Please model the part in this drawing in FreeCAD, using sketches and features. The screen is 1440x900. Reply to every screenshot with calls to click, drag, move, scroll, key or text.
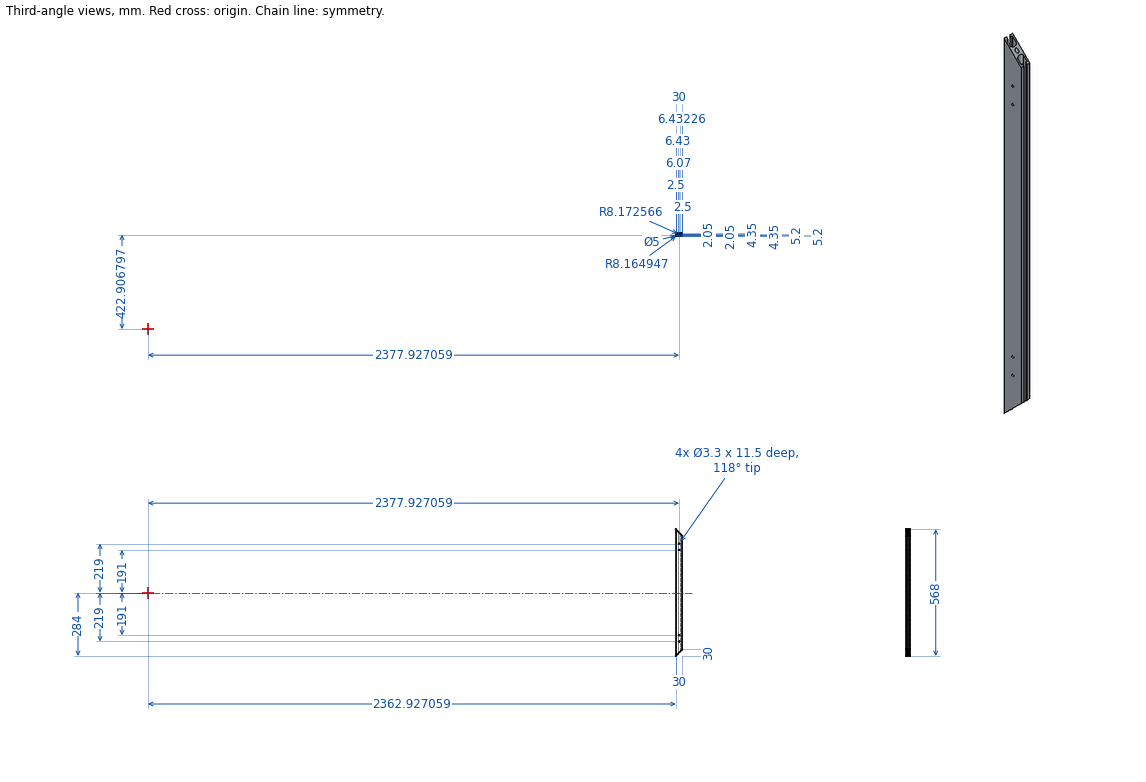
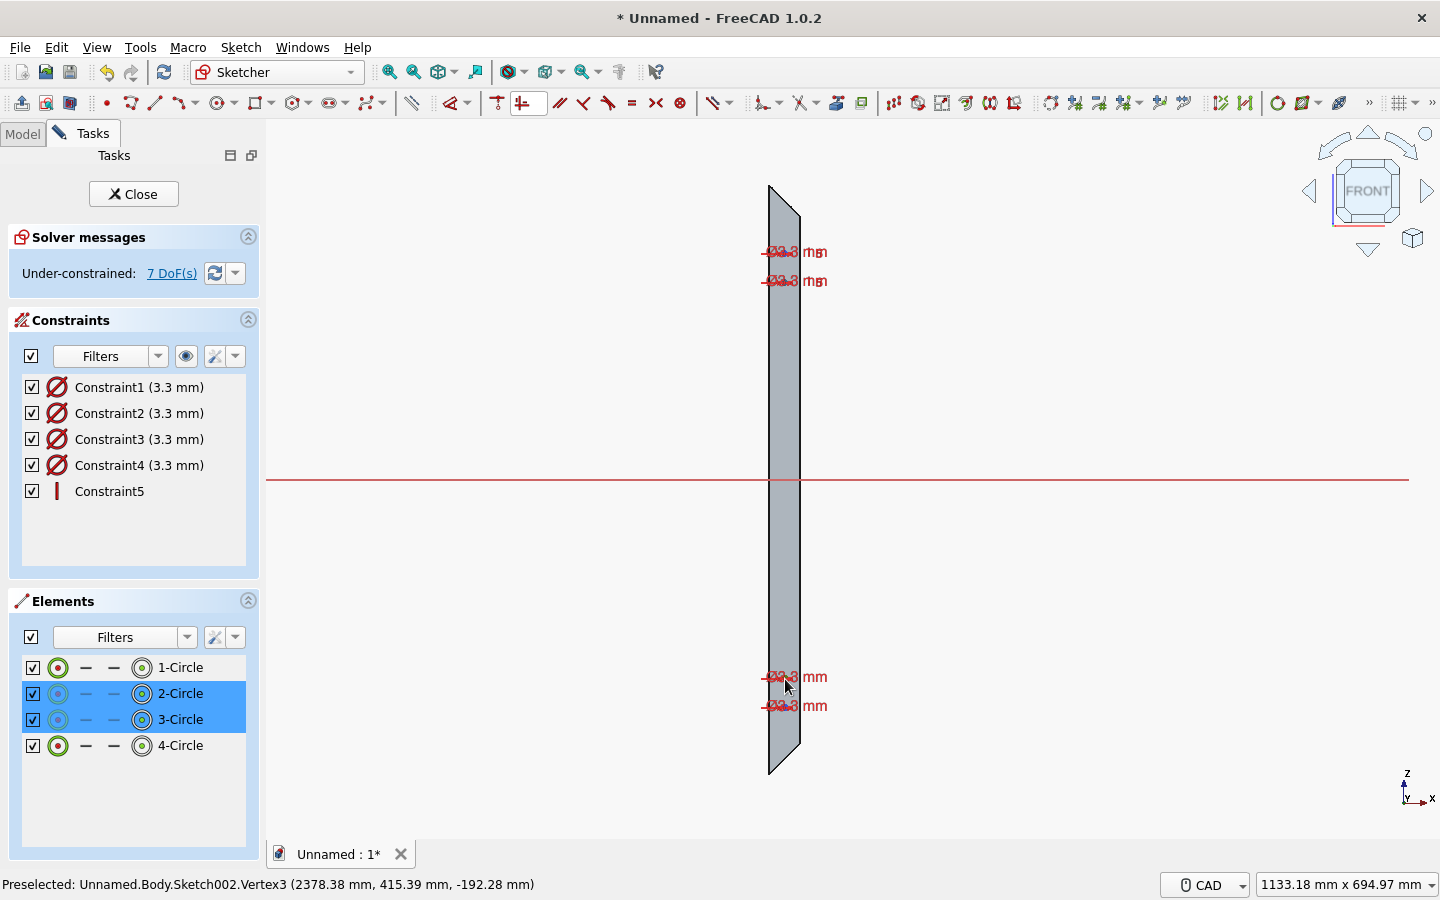
click(542, 104)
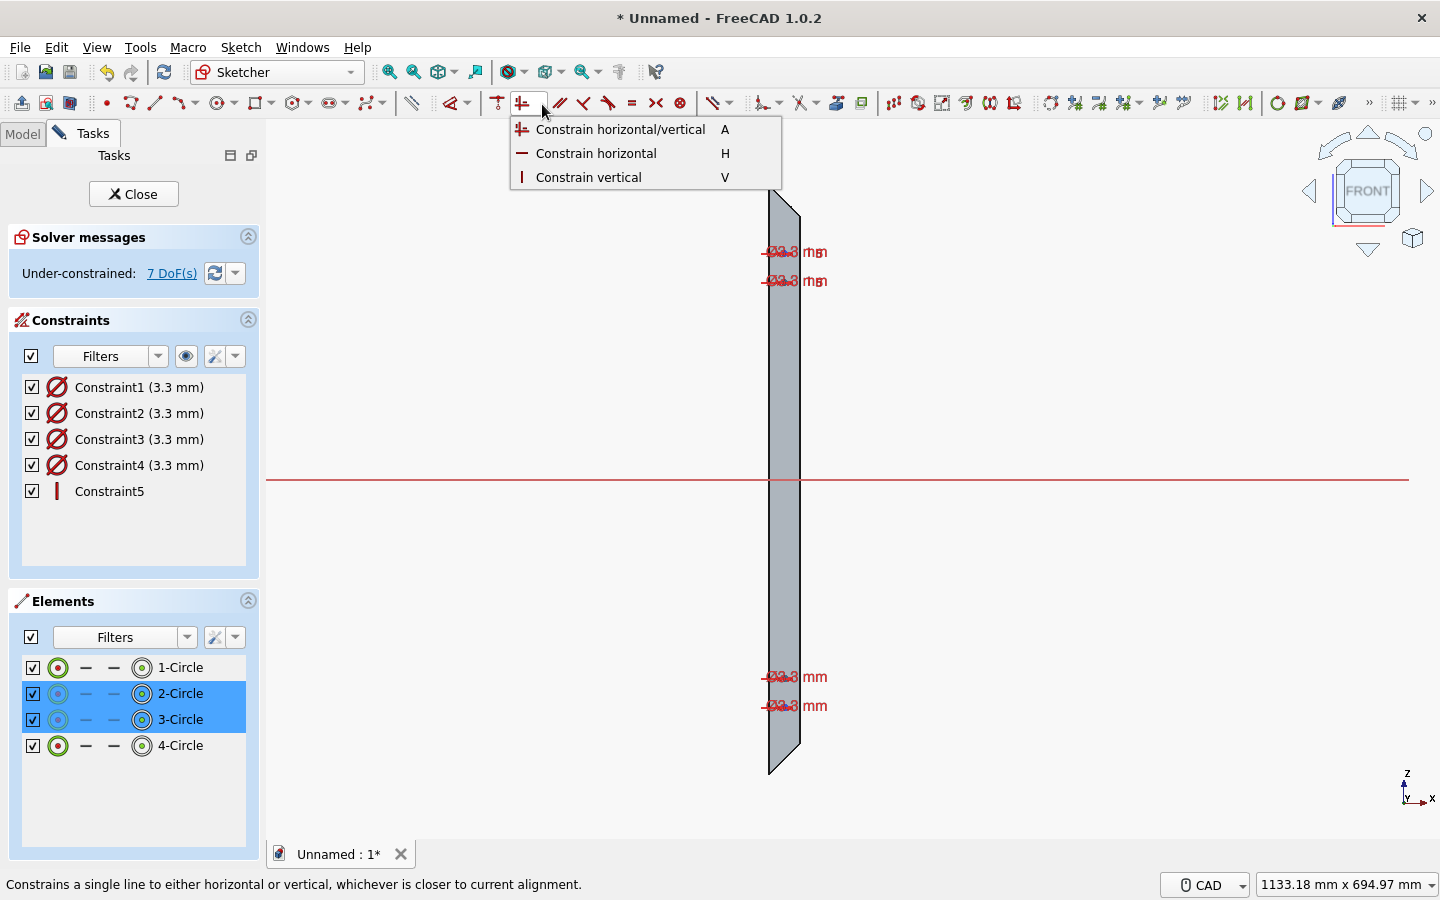
click(646, 177)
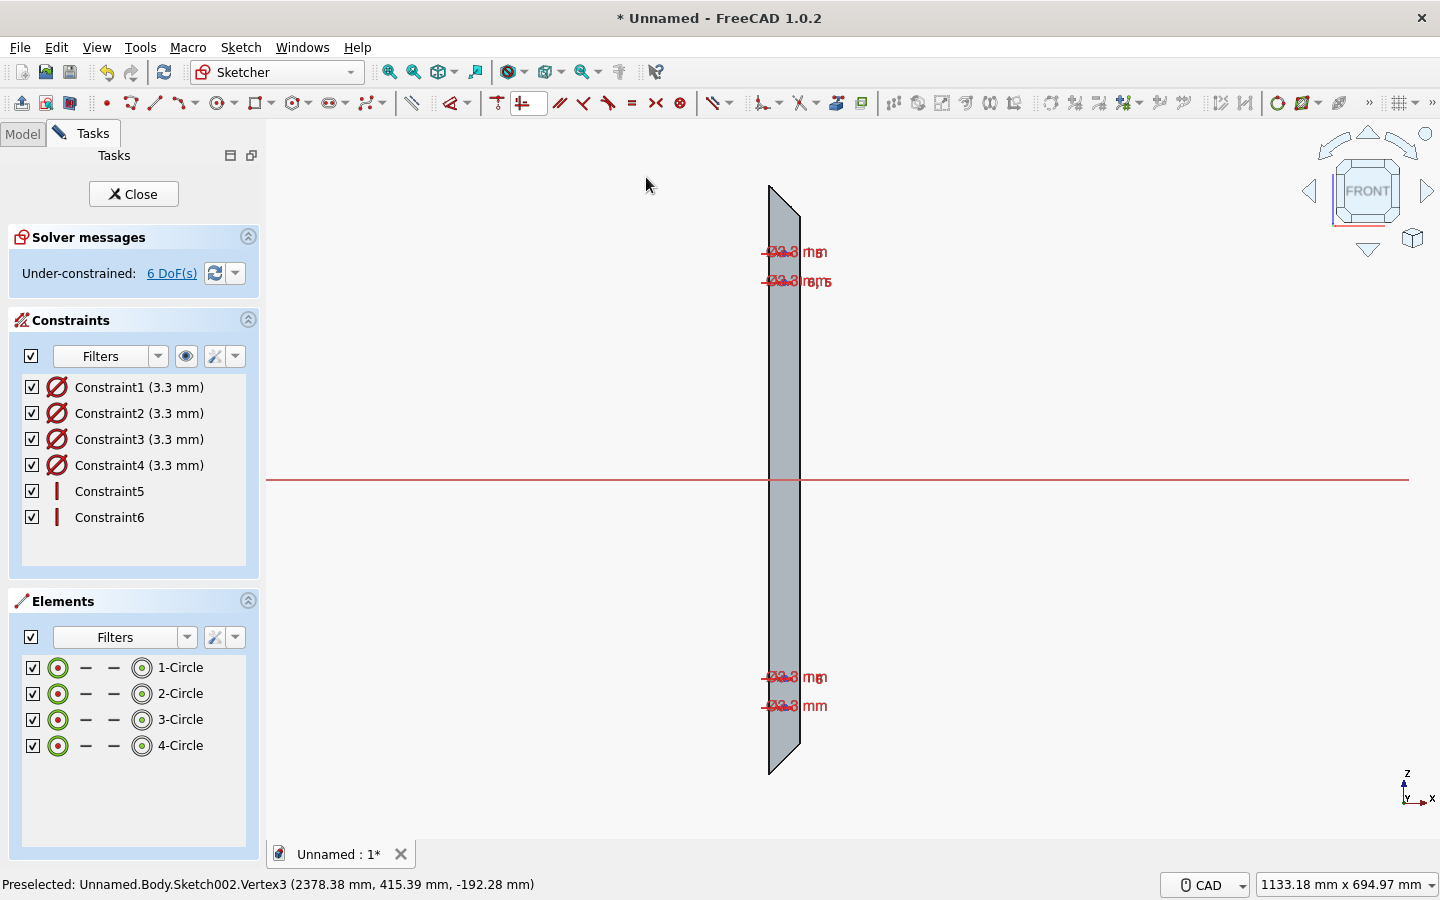
click(785, 679)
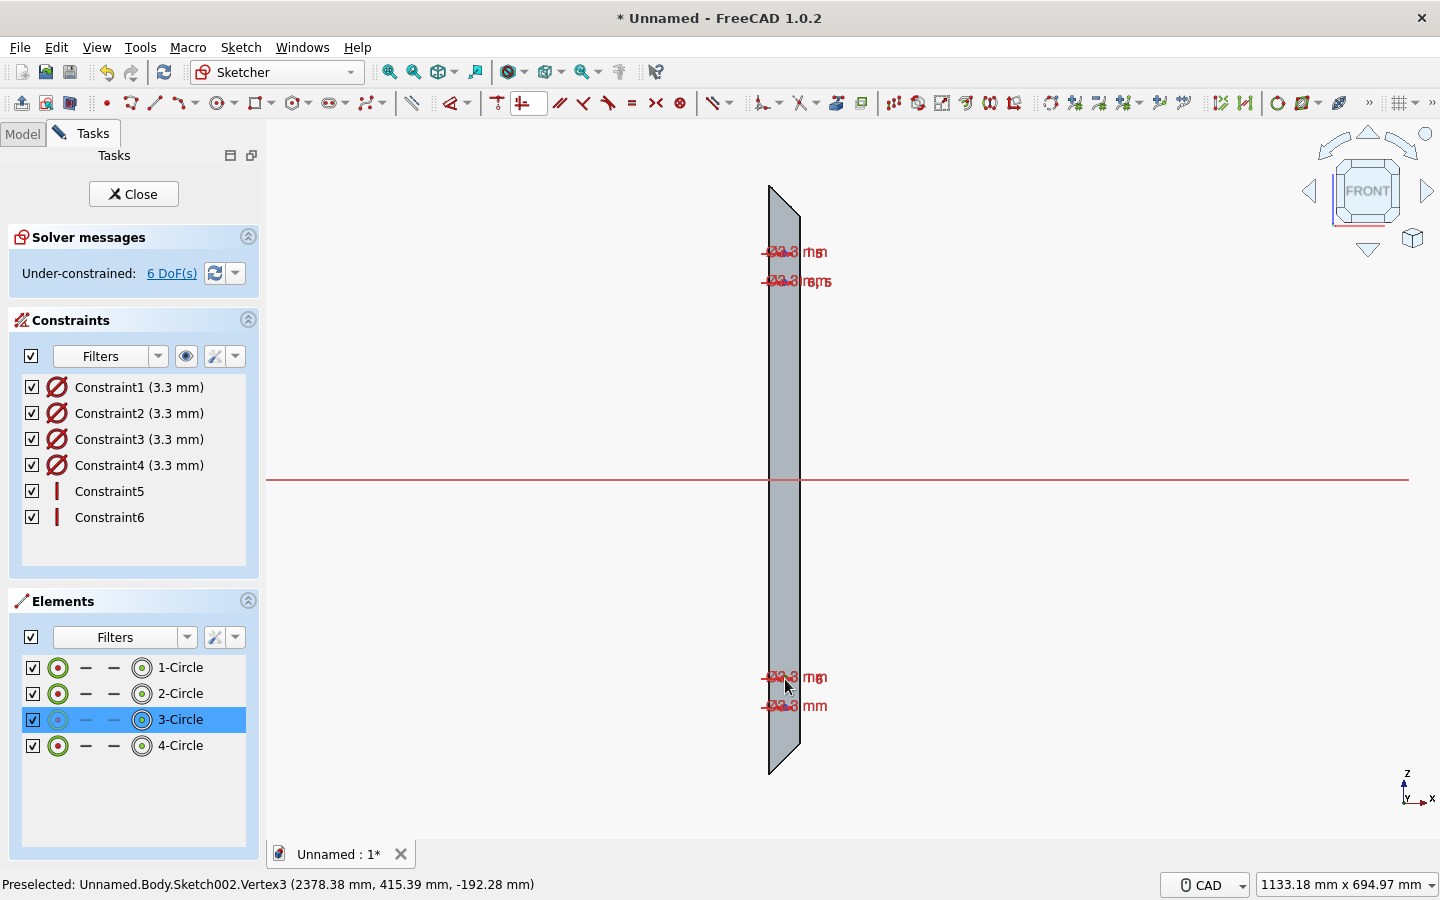
click(785, 708)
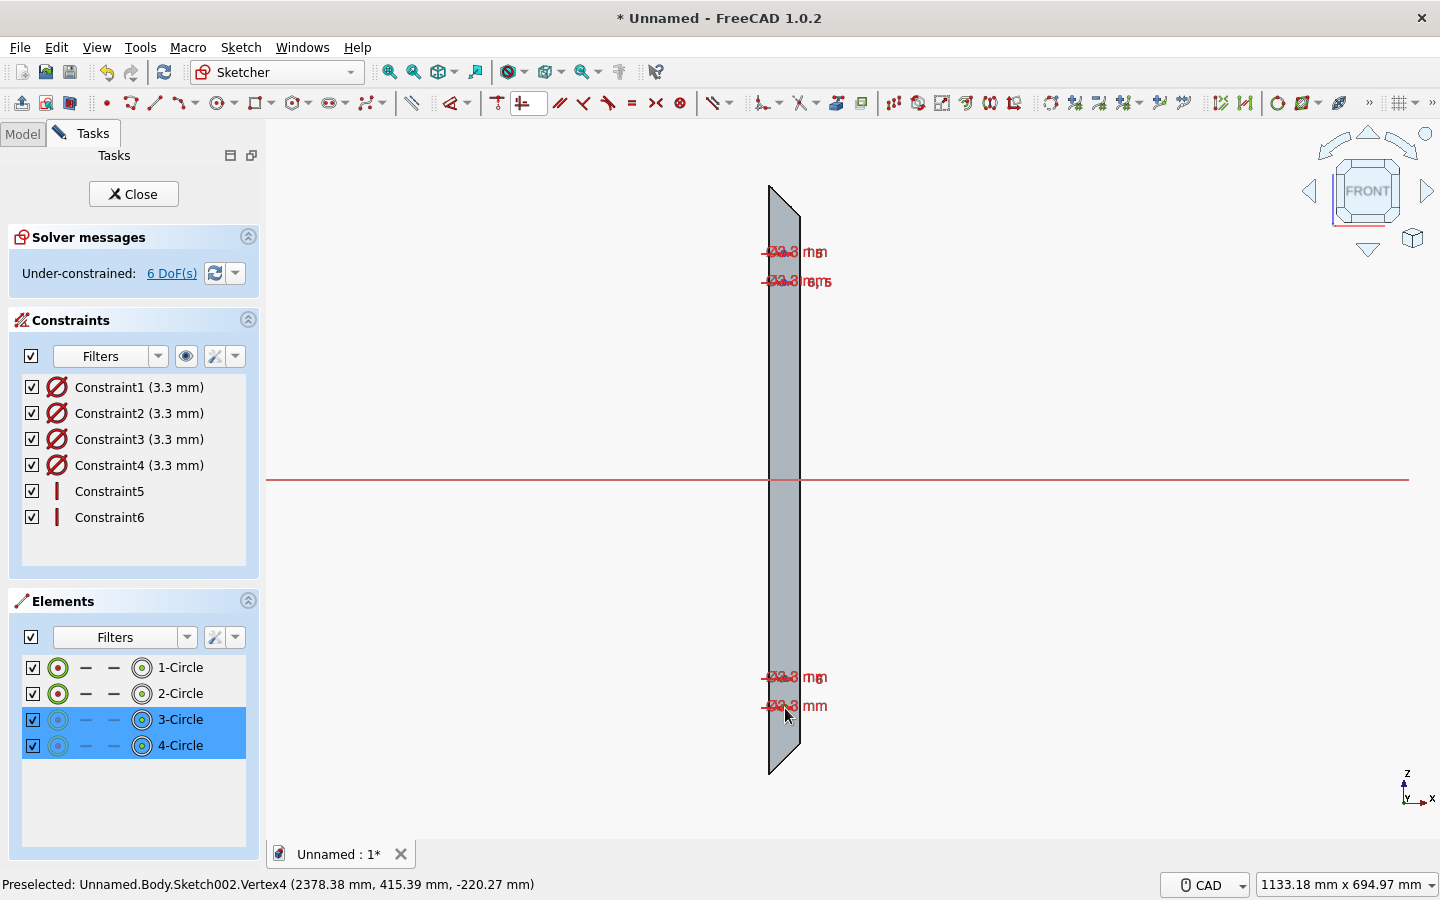
key(v)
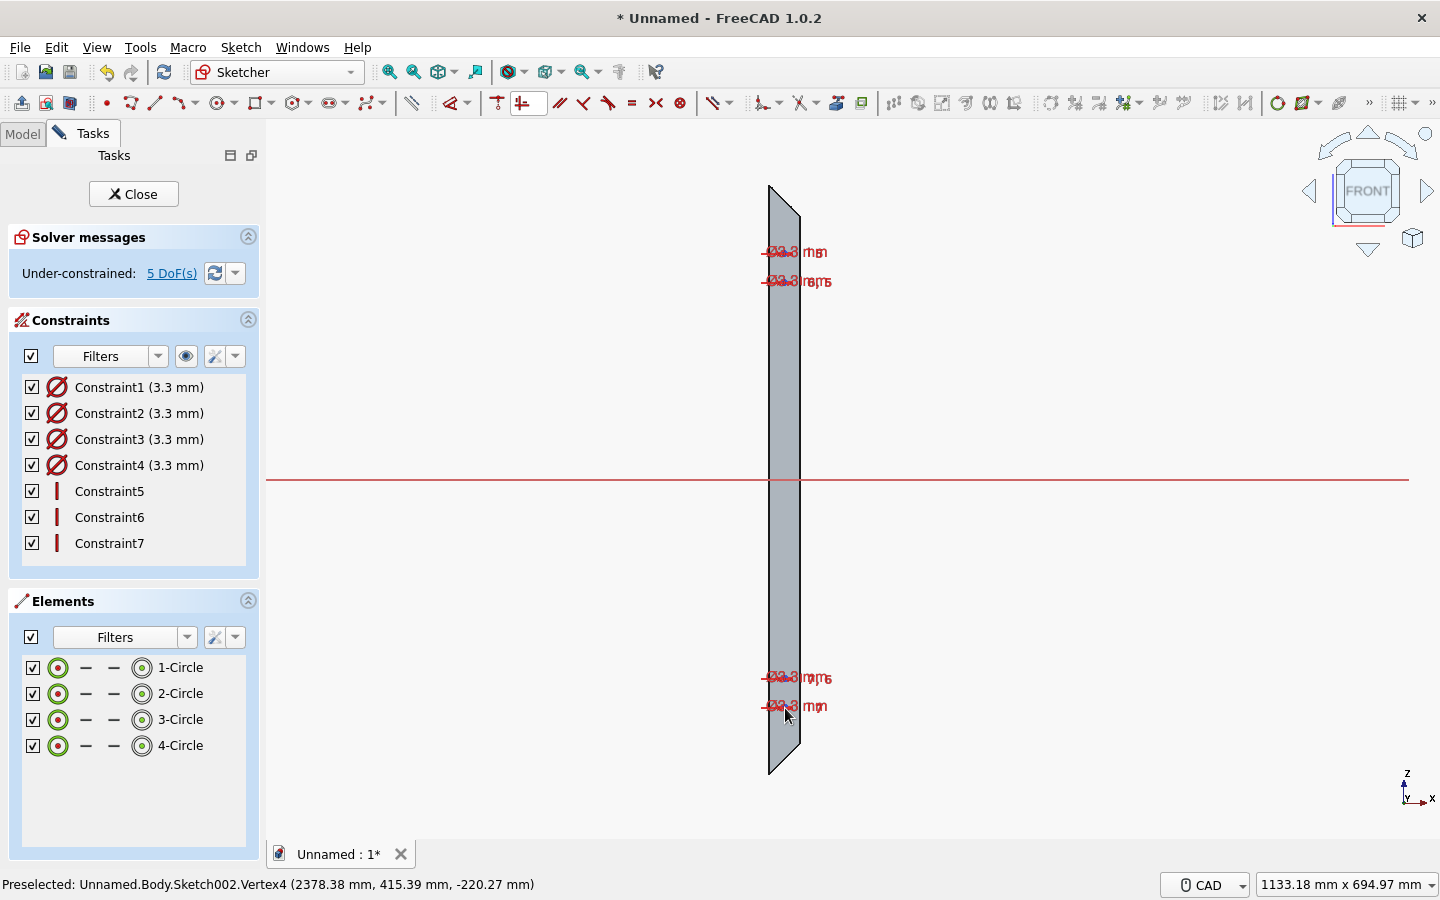
click(450, 104)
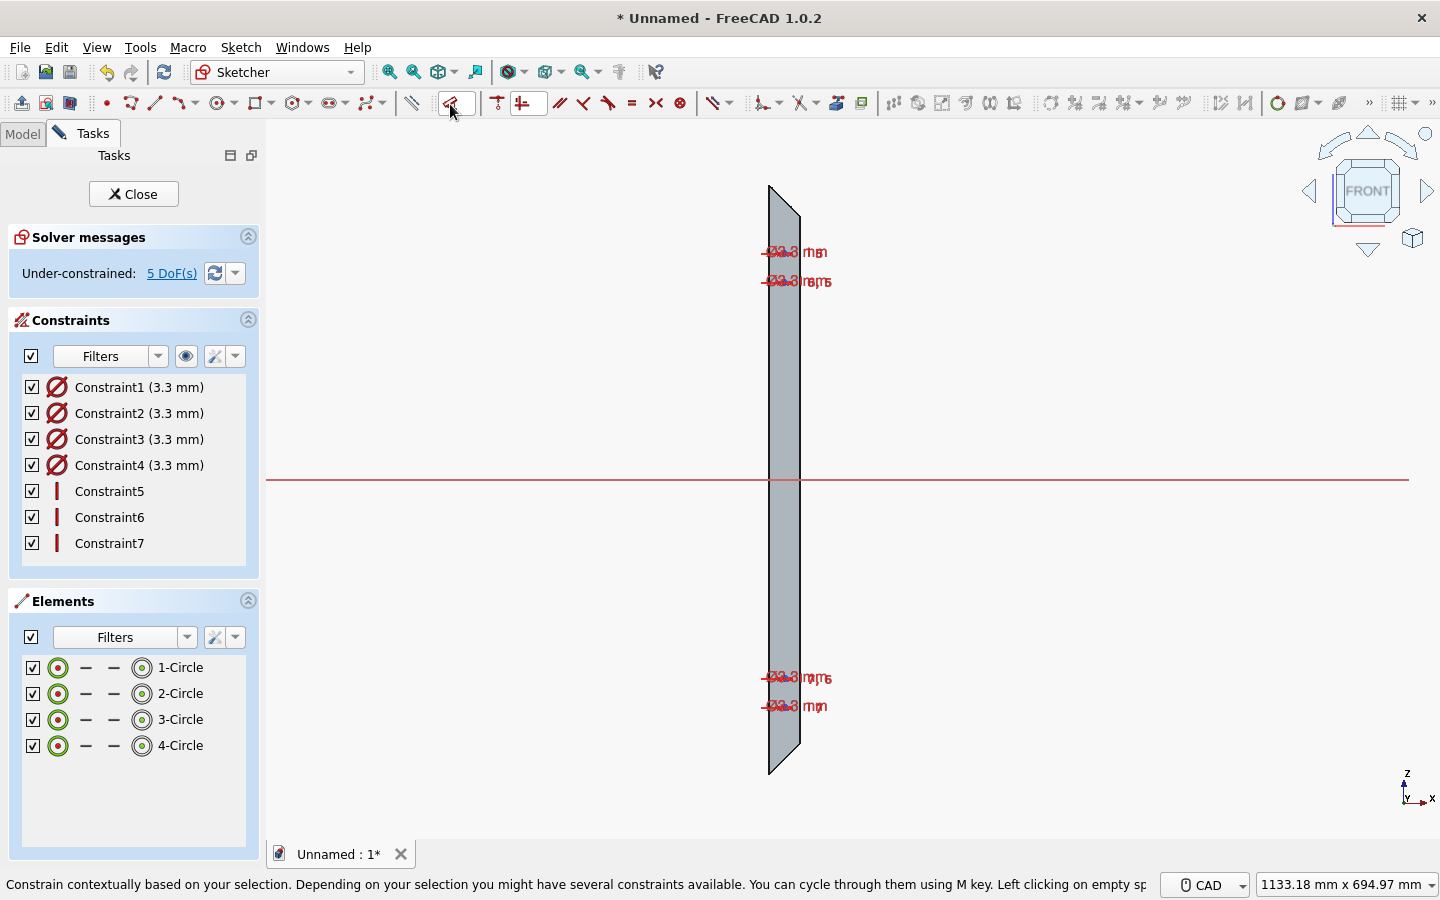
click(785, 254)
click(819, 367)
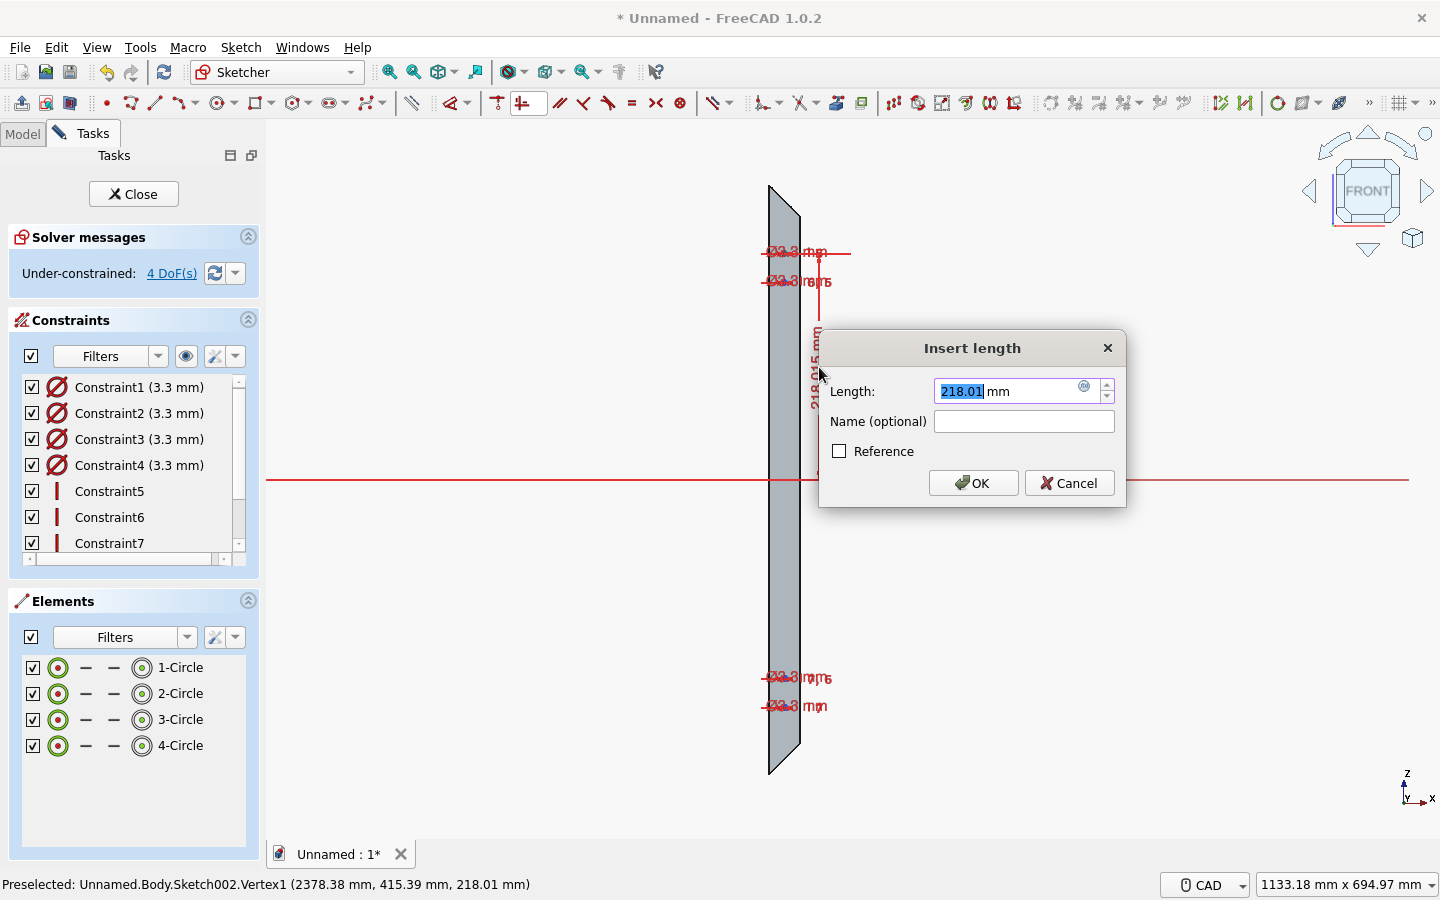
text(219)
key(Return)